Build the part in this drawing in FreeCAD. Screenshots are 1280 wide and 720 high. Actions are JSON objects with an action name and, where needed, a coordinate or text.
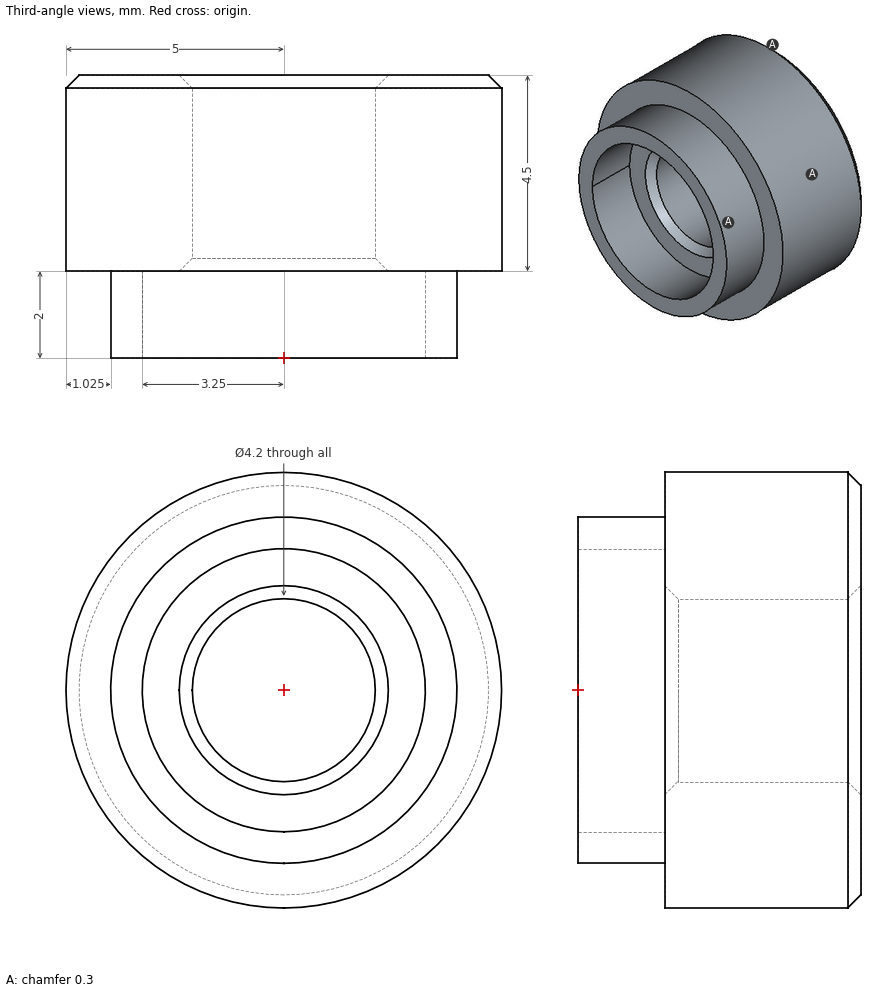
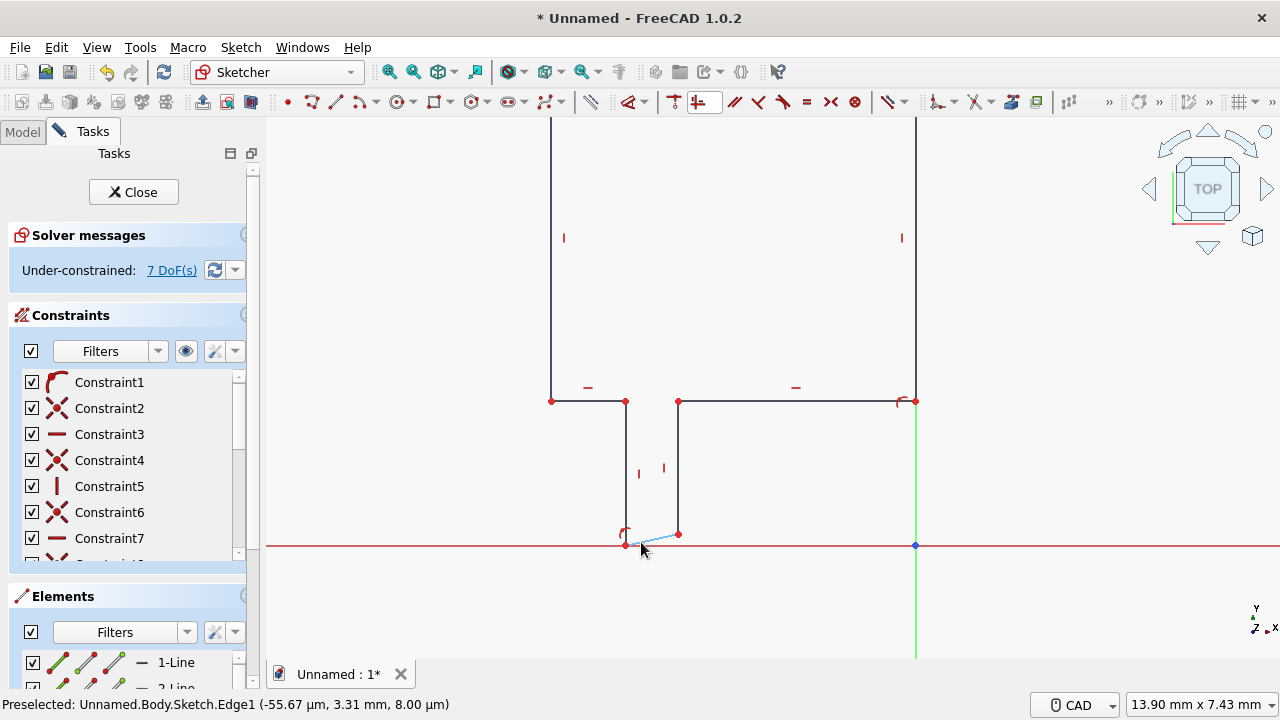
{"action": "left_click", "coordinate": [642, 542]}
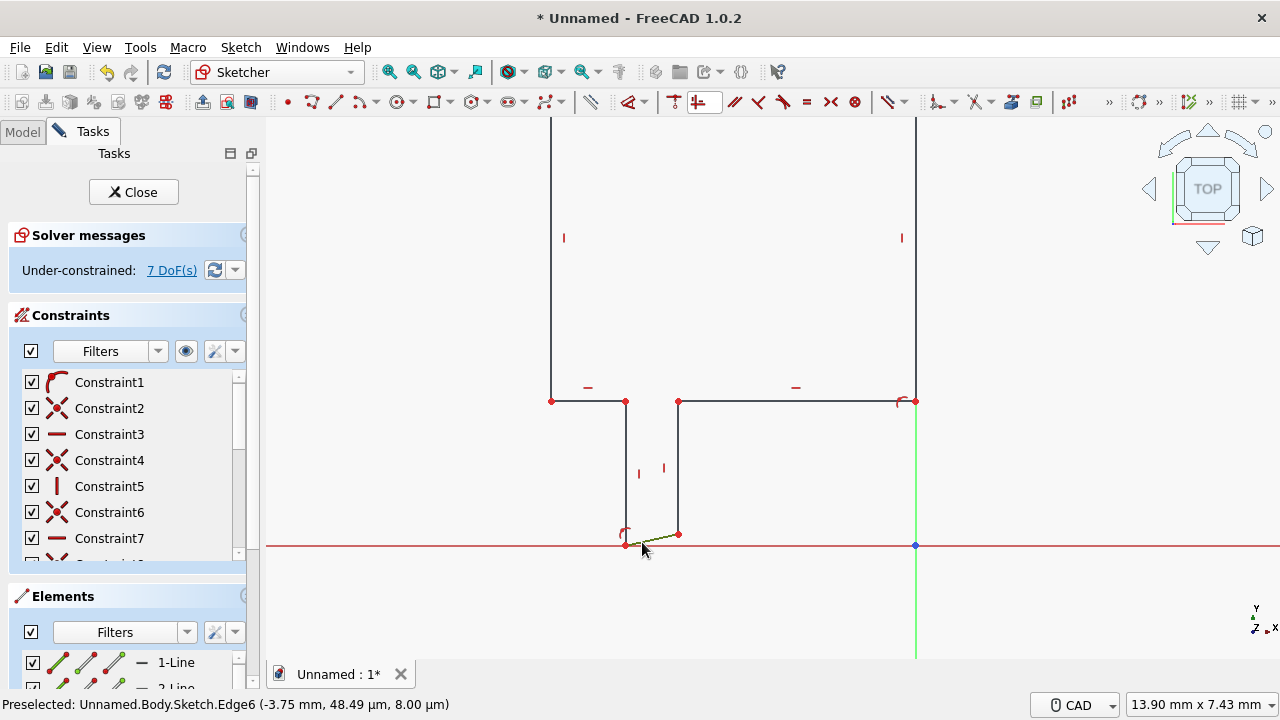
{"action": "left_click", "coordinate": [716, 102]}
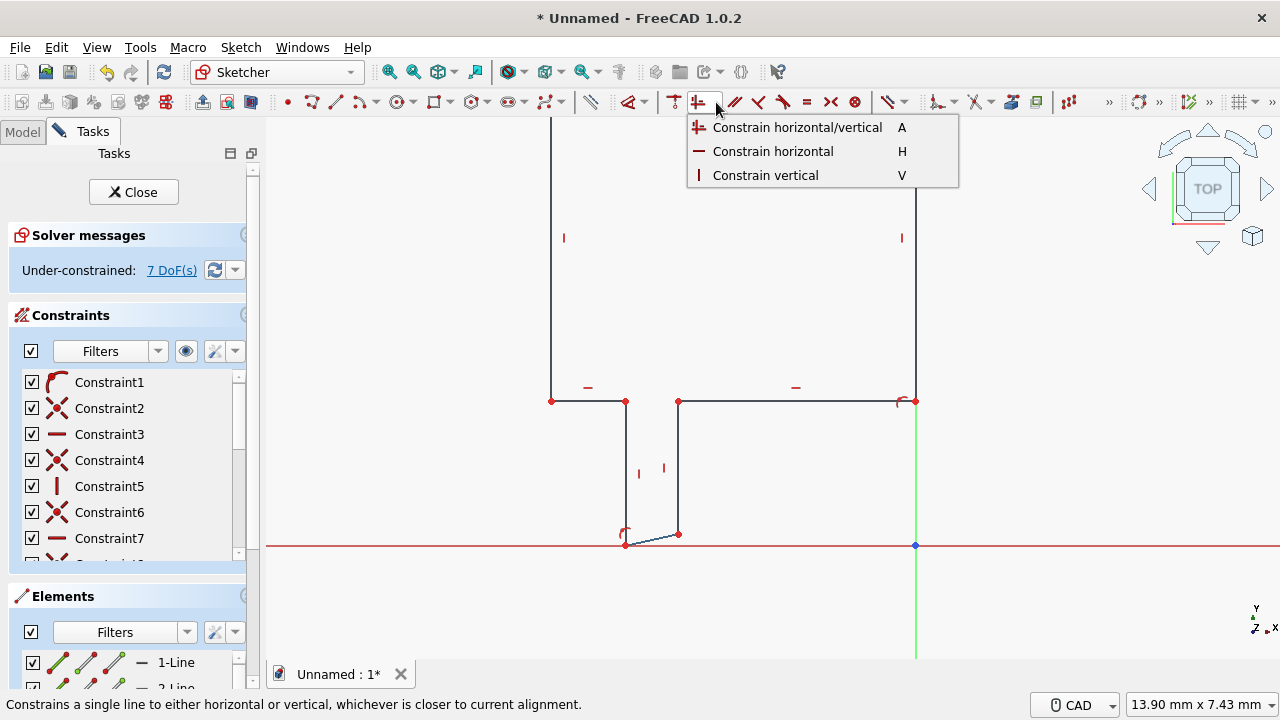
{"action": "left_click", "coordinate": [823, 151]}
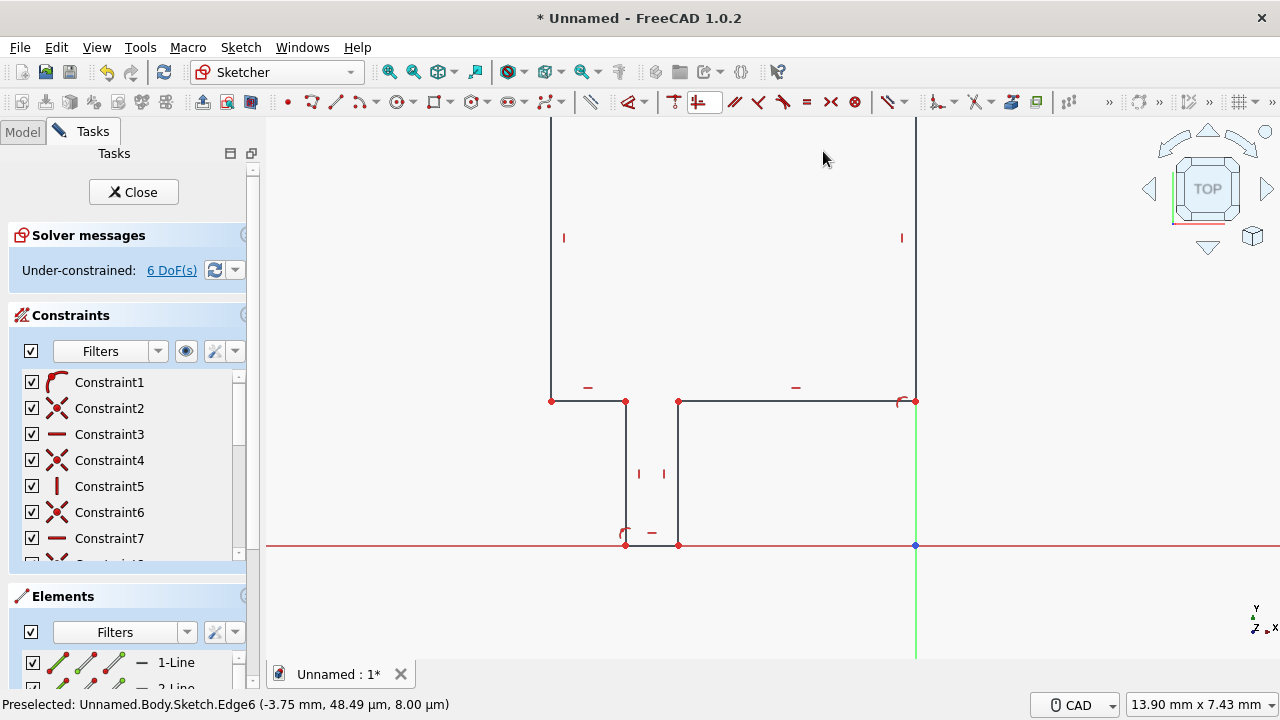
{"action": "left_click", "coordinate": [628, 102]}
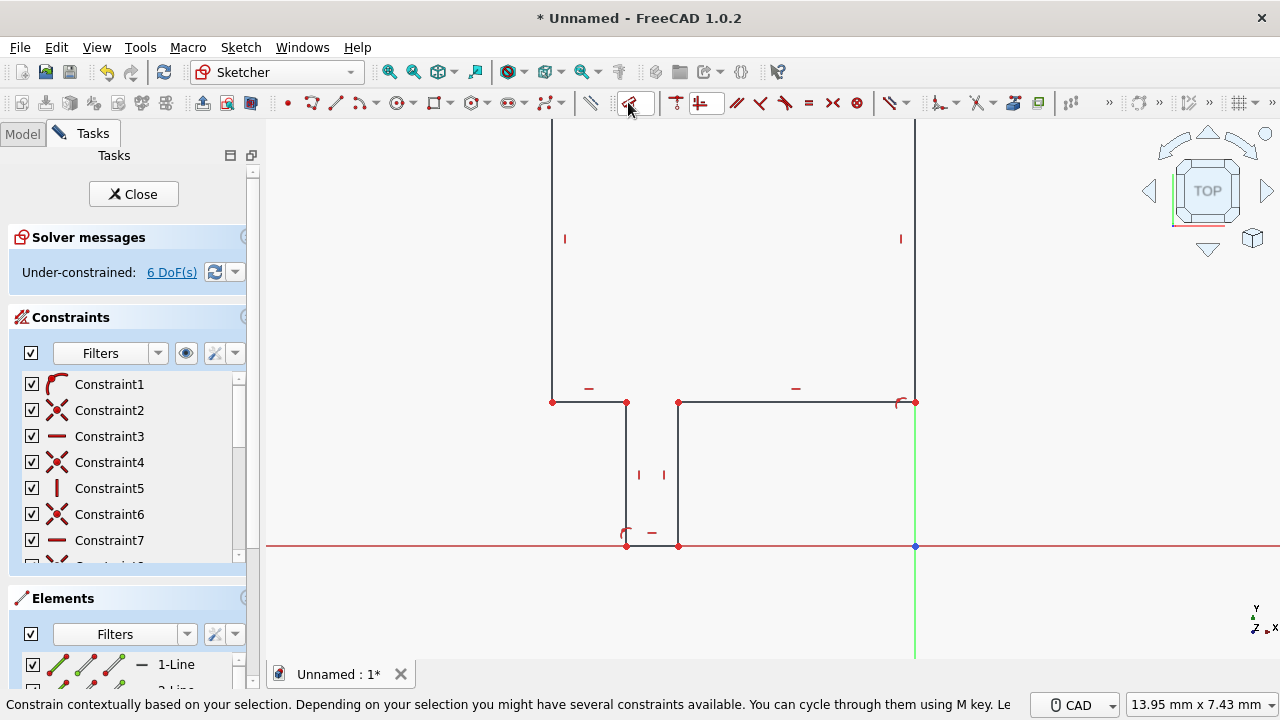
{"action": "scroll", "coordinate": [646, 550], "scroll_direction": "down", "scroll_amount": 2}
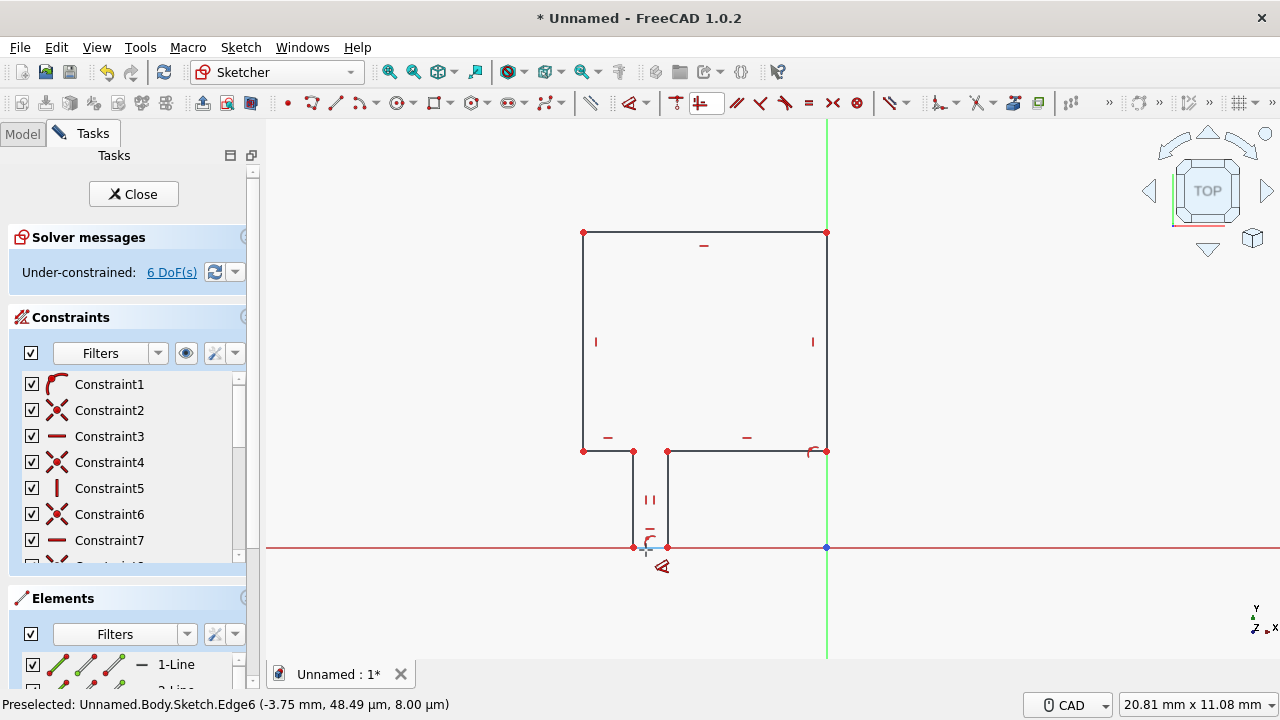
{"action": "left_click", "coordinate": [754, 232]}
{"action": "left_click", "coordinate": [705, 198]}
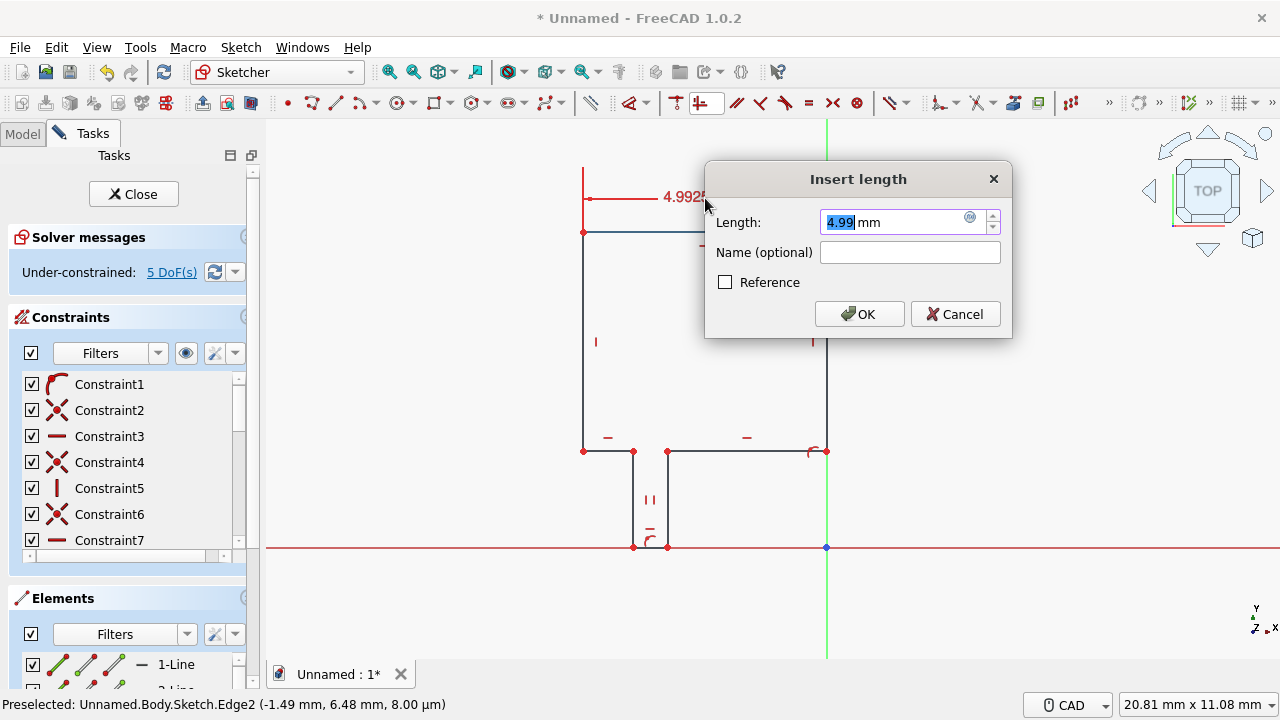
{"action": "type", "text": "5"}
{"action": "key", "text": "Return"}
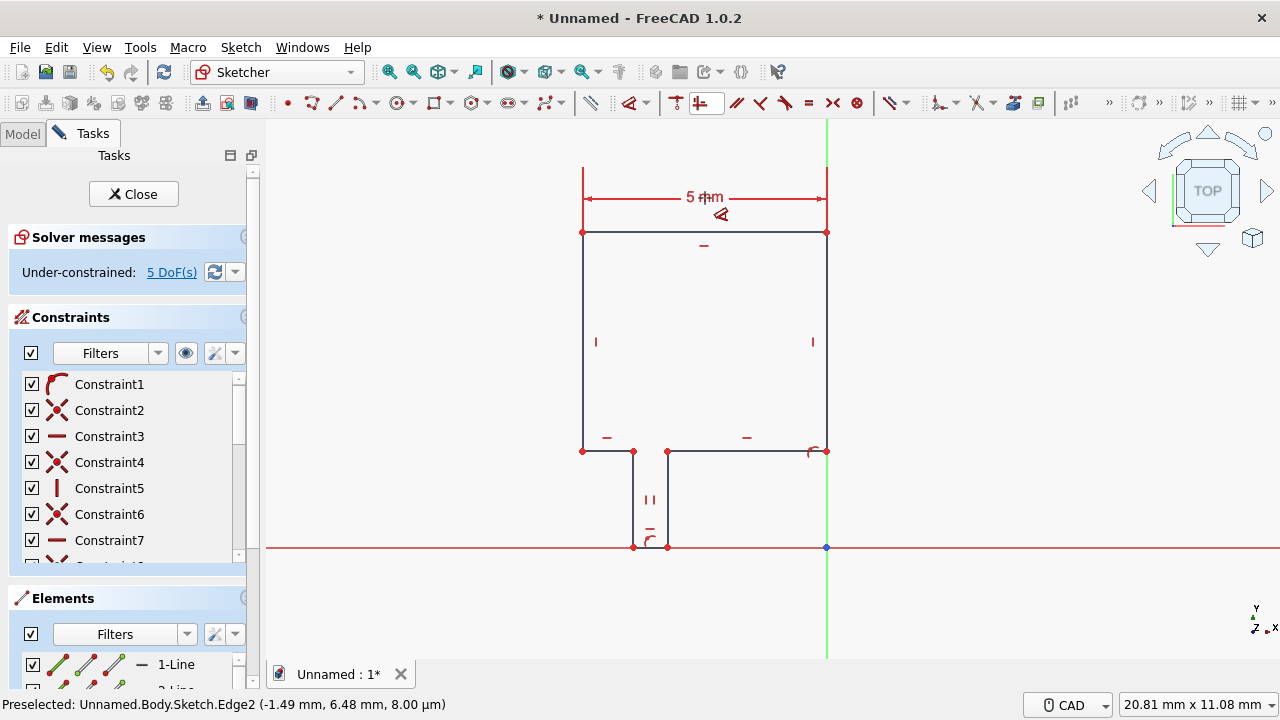
{"action": "left_click", "coordinate": [633, 480]}
{"action": "left_click", "coordinate": [599, 499]}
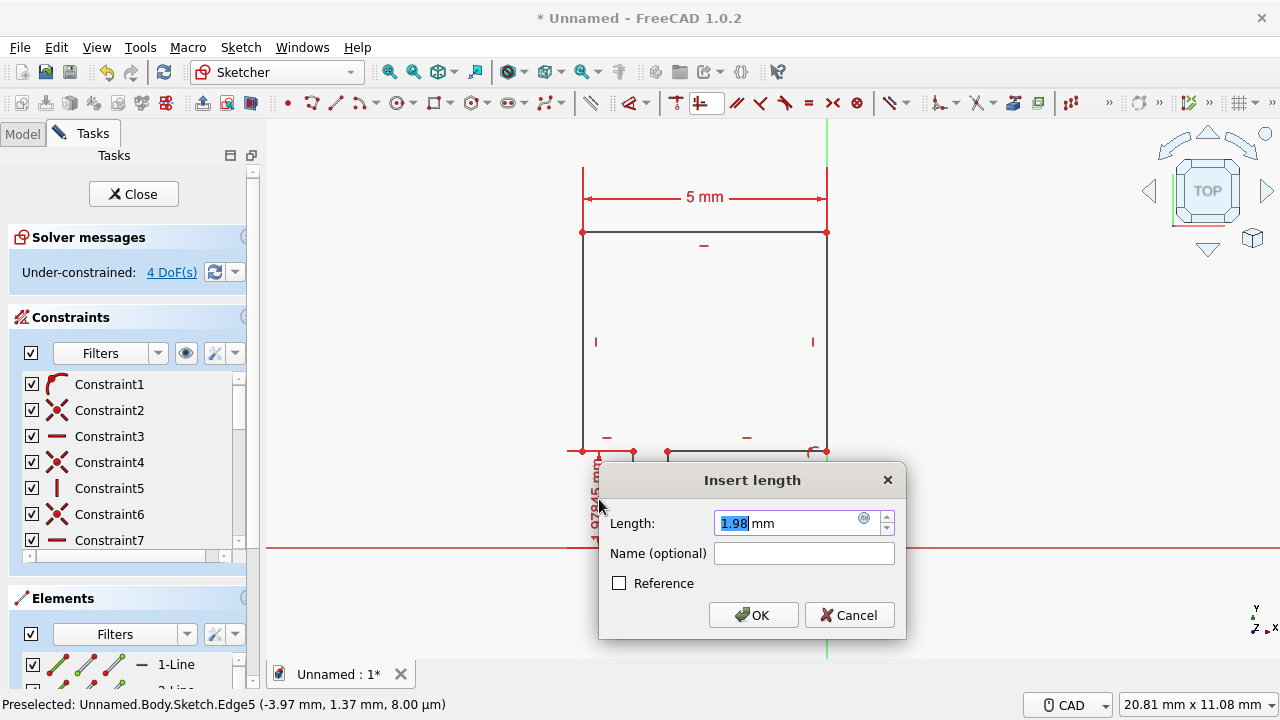
{"action": "type", "text": "2"}
{"action": "key", "text": "Return"}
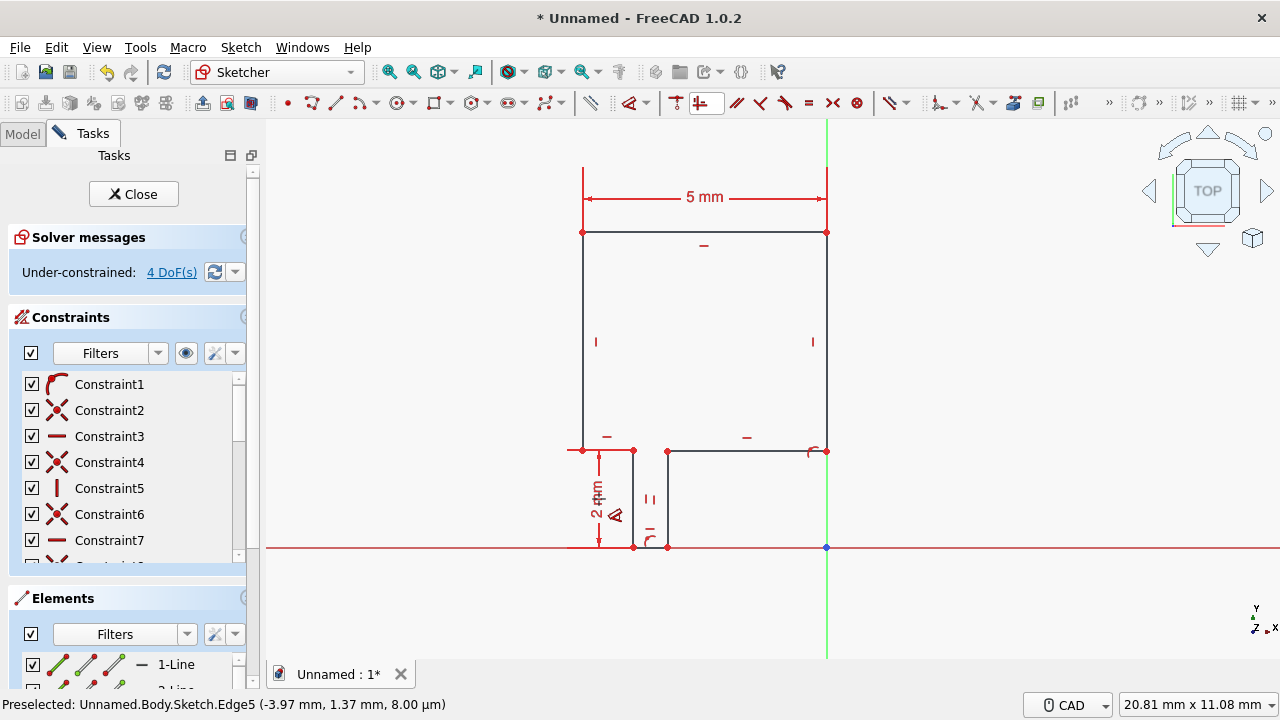
{"action": "left_click", "coordinate": [668, 519]}
{"action": "left_click", "coordinate": [702, 499]}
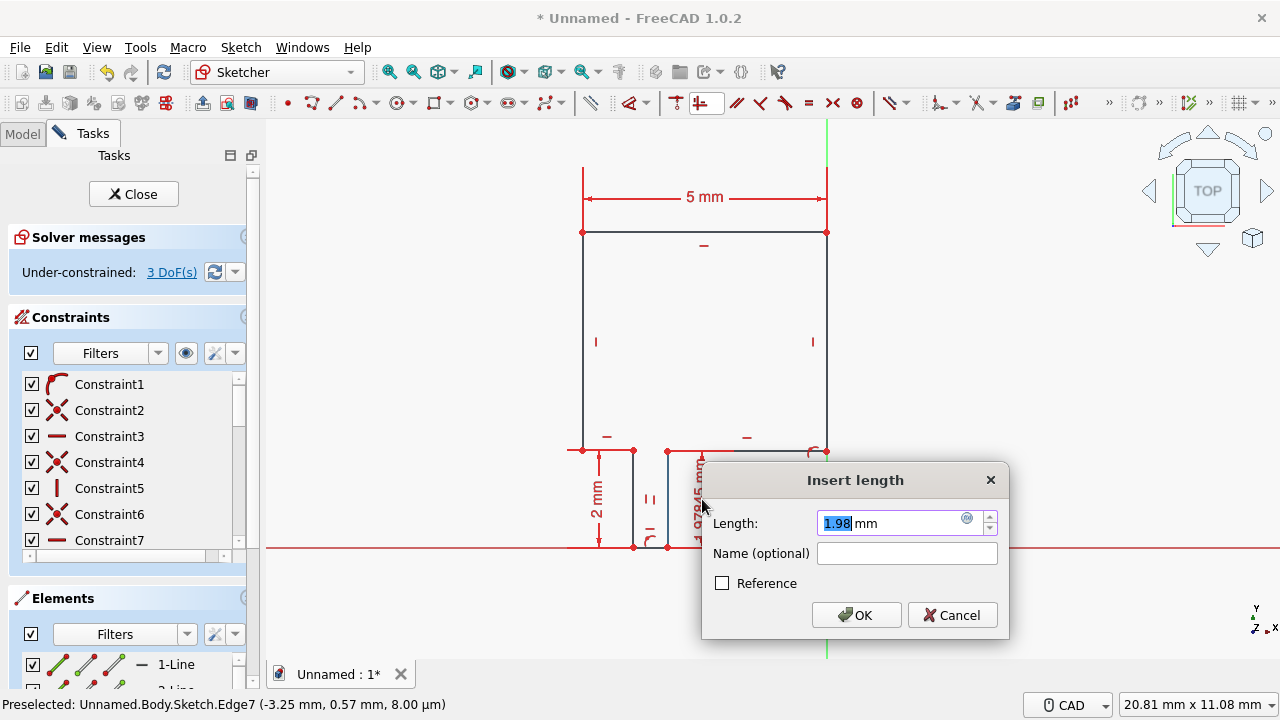
{"action": "type", "text": "2"}
{"action": "key", "text": "Return"}